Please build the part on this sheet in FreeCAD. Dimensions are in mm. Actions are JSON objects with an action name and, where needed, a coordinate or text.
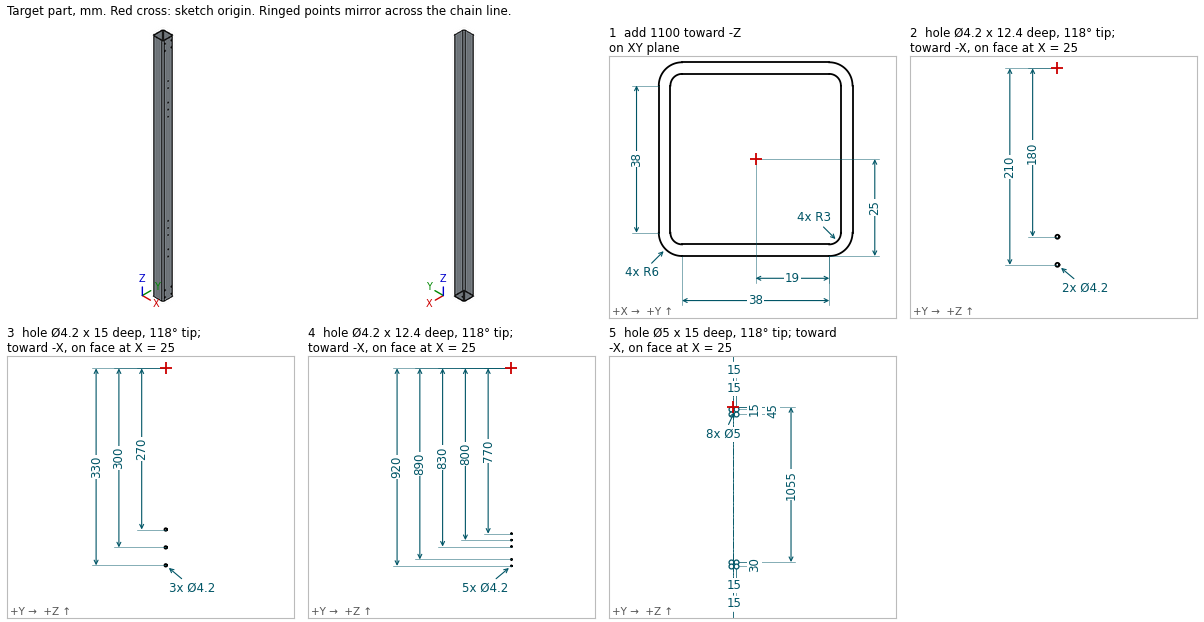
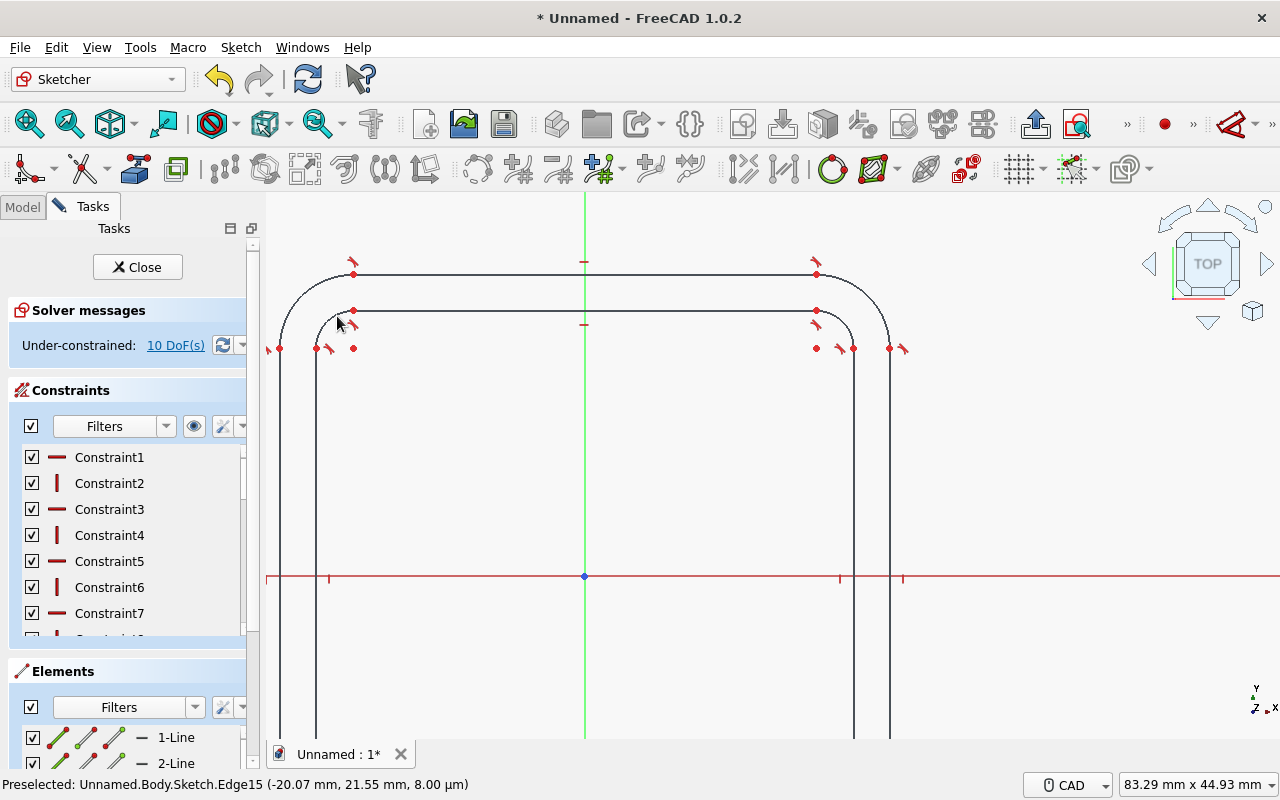
{"action": "scroll", "coordinate": [850, 330], "scroll_direction": "down", "scroll_amount": 3}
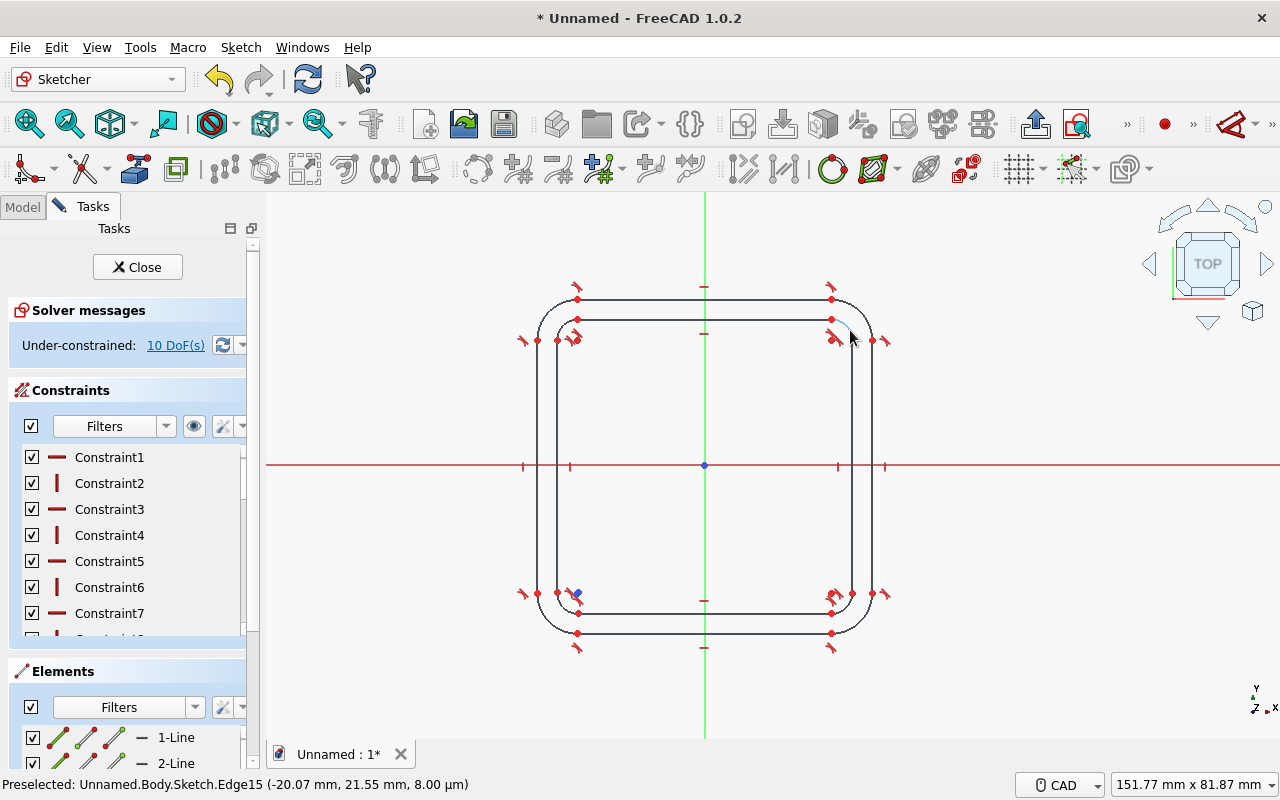
{"action": "left_click", "coordinate": [542, 612]}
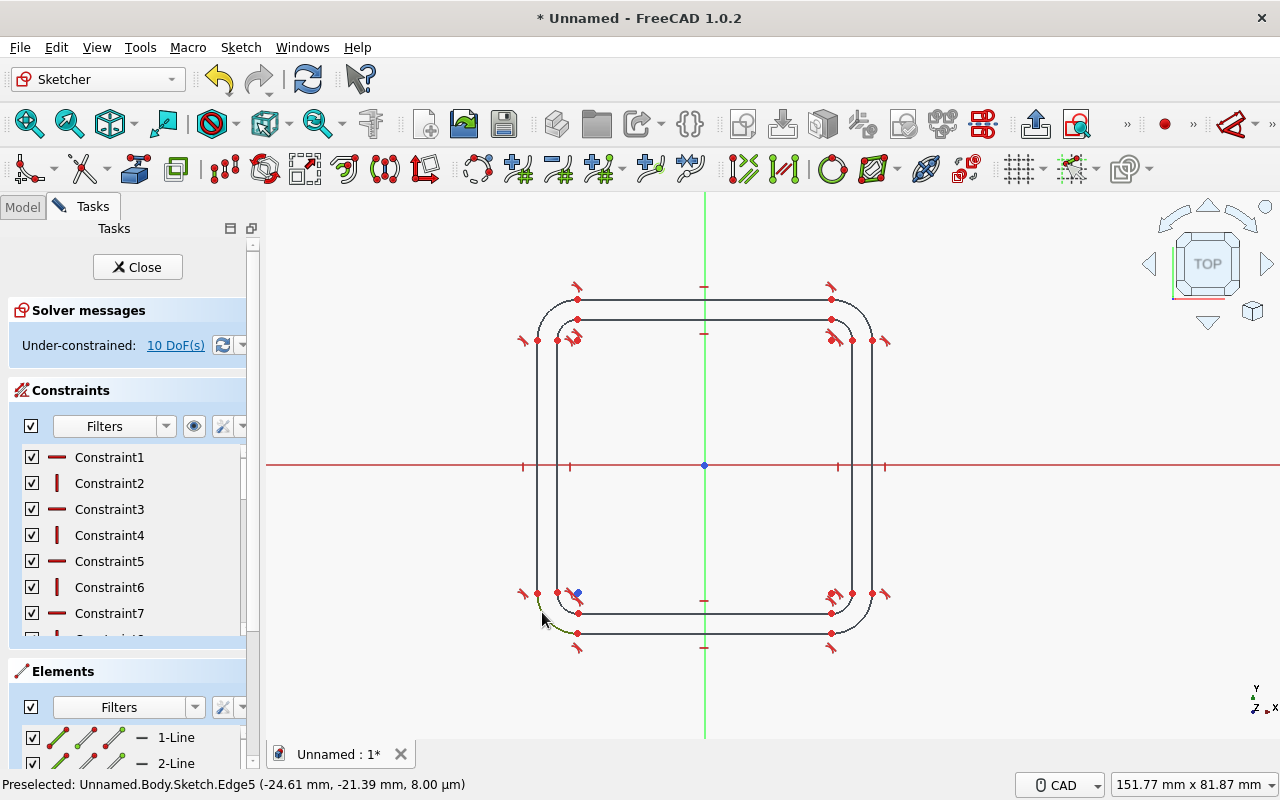
{"action": "left_click", "coordinate": [559, 304]}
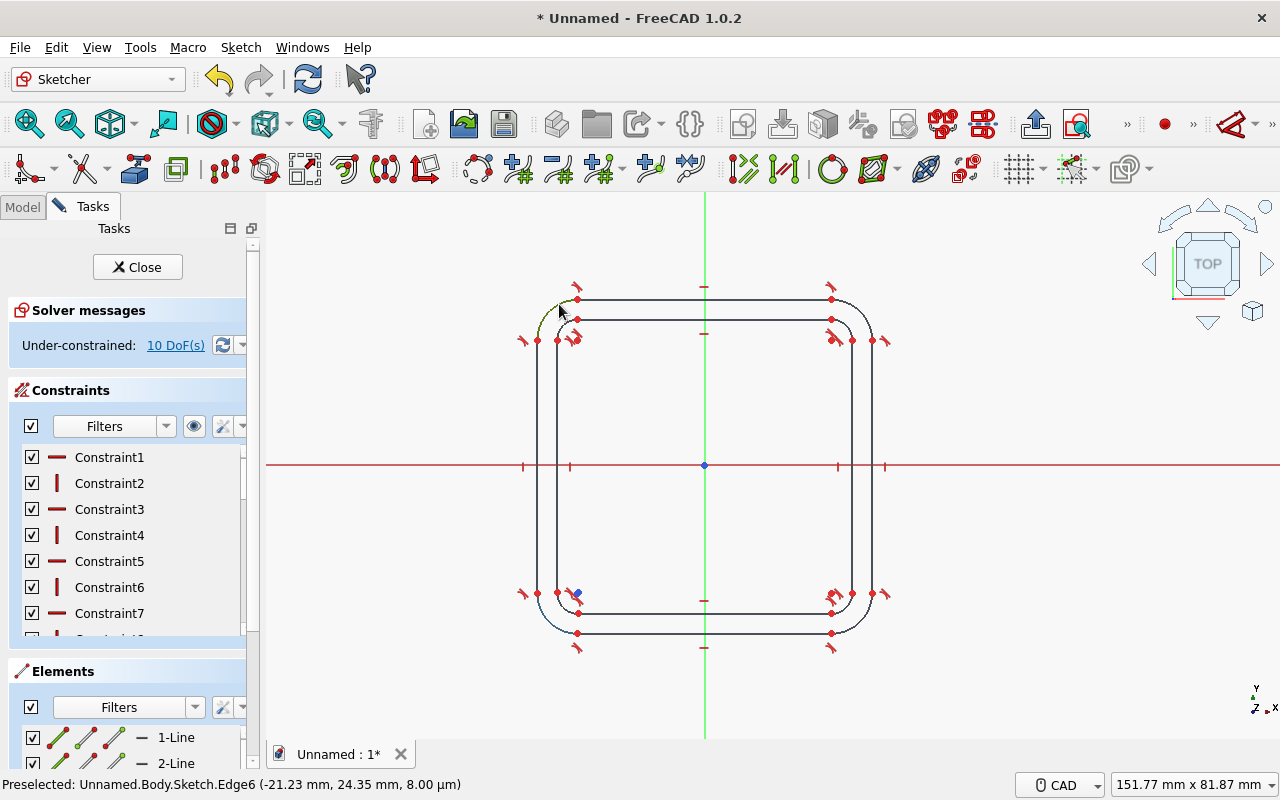
{"action": "left_click", "coordinate": [868, 322]}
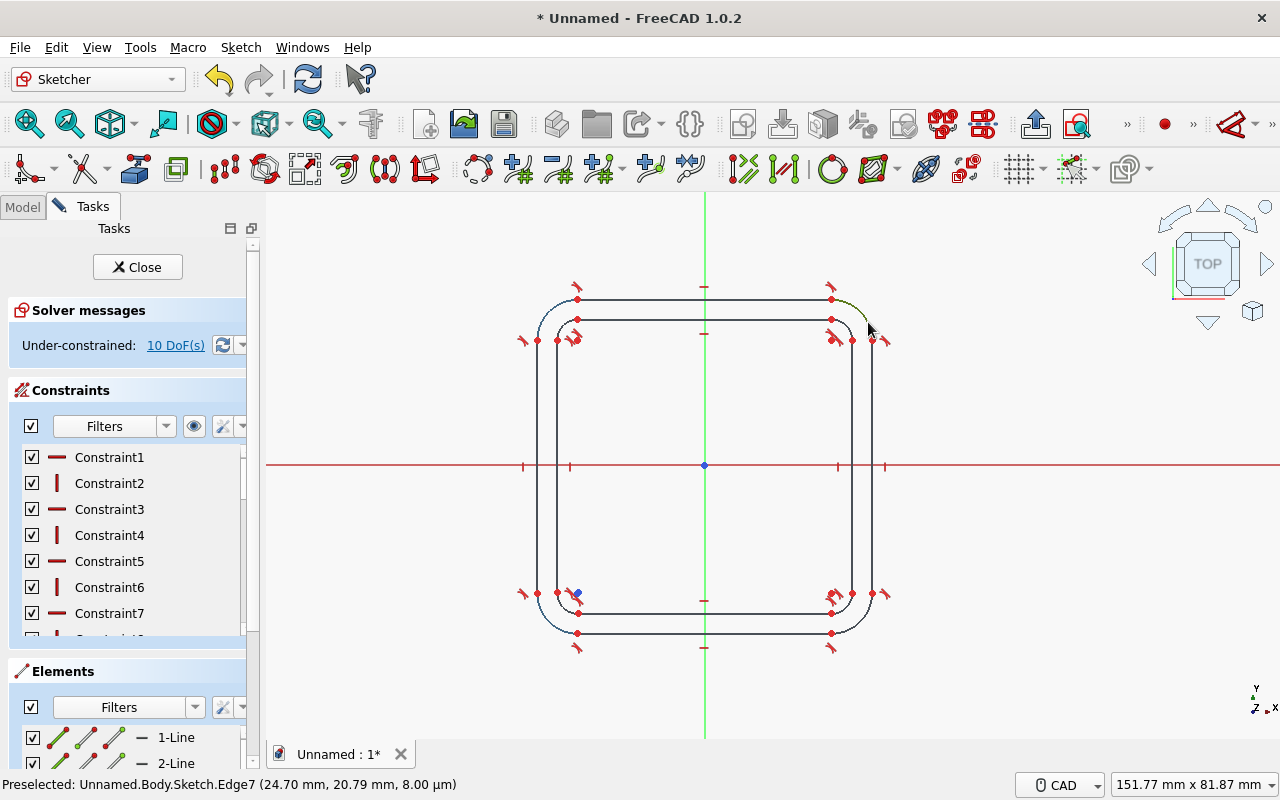
{"action": "left_click", "coordinate": [850, 629]}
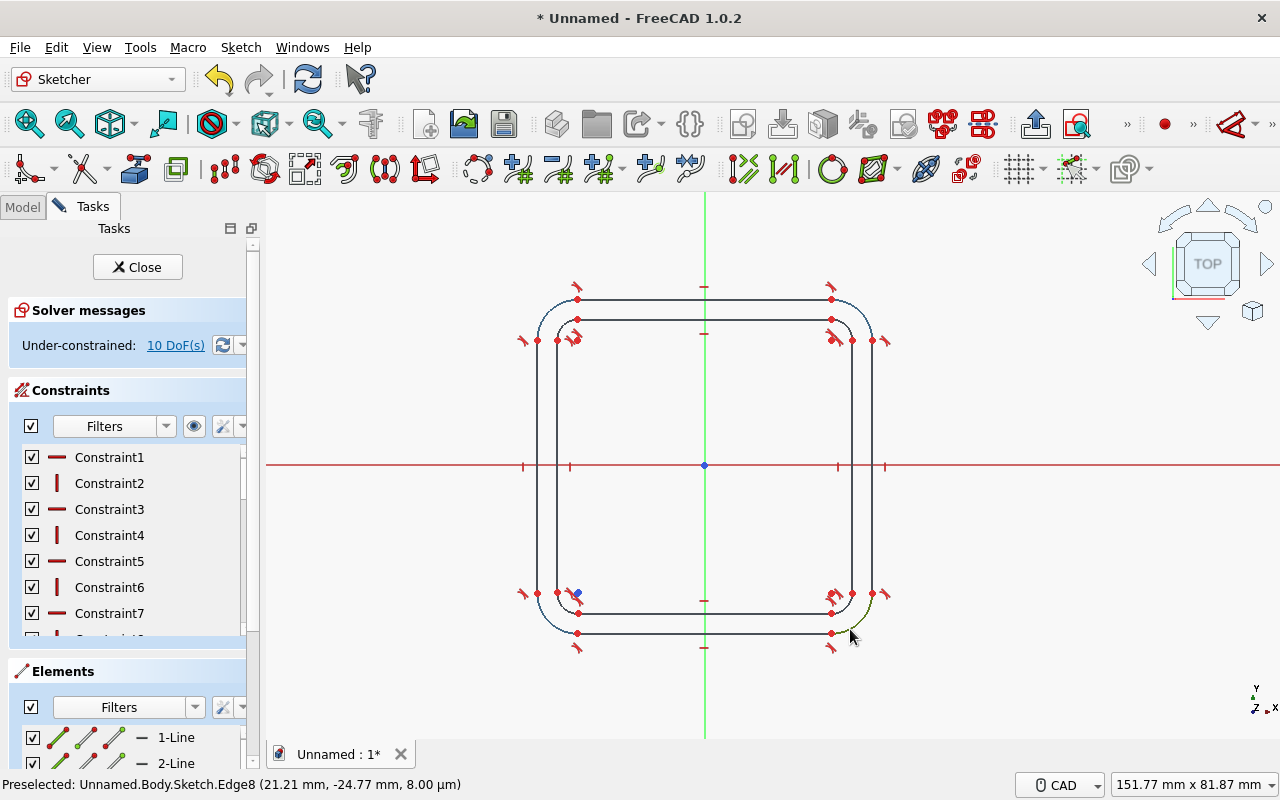
{"action": "key", "text": "e"}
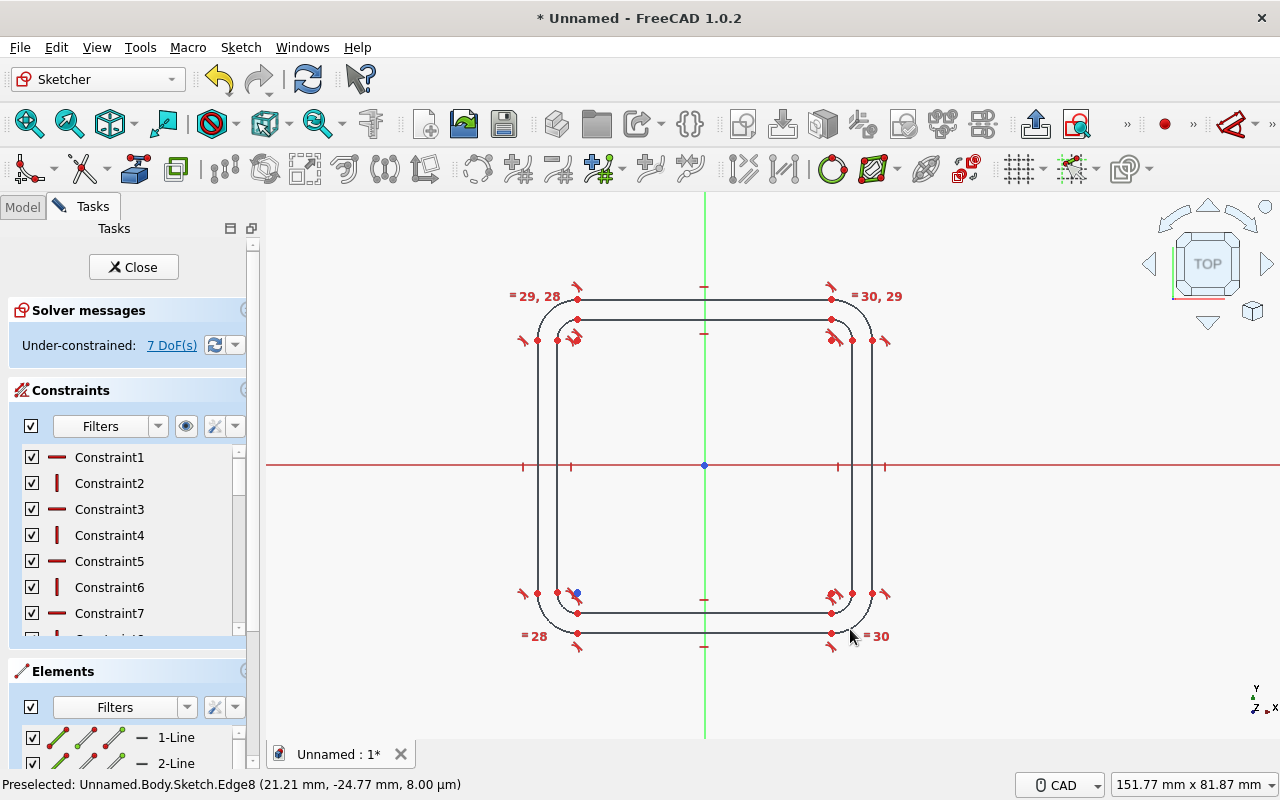
{"action": "scroll", "coordinate": [841, 611], "scroll_direction": "up", "scroll_amount": 2}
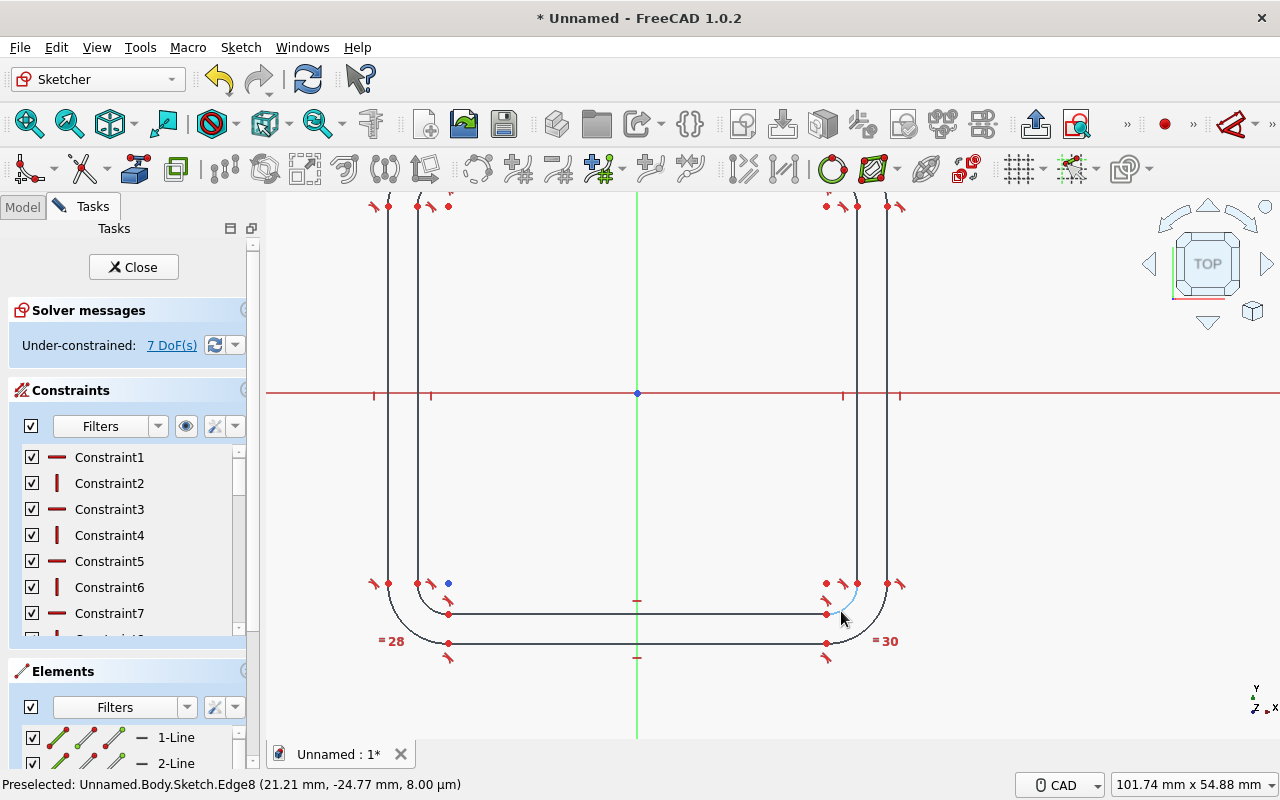
{"action": "left_click", "coordinate": [841, 611]}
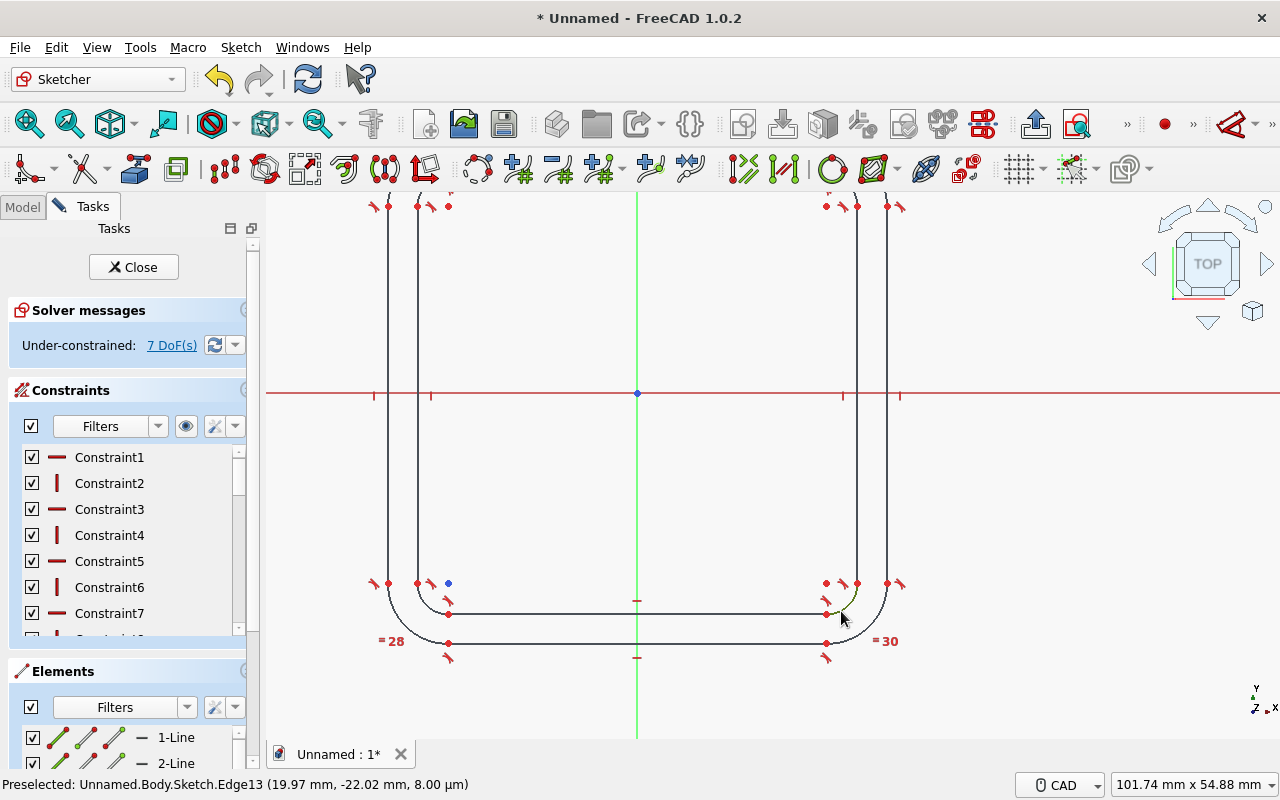
{"action": "left_click", "coordinate": [421, 598]}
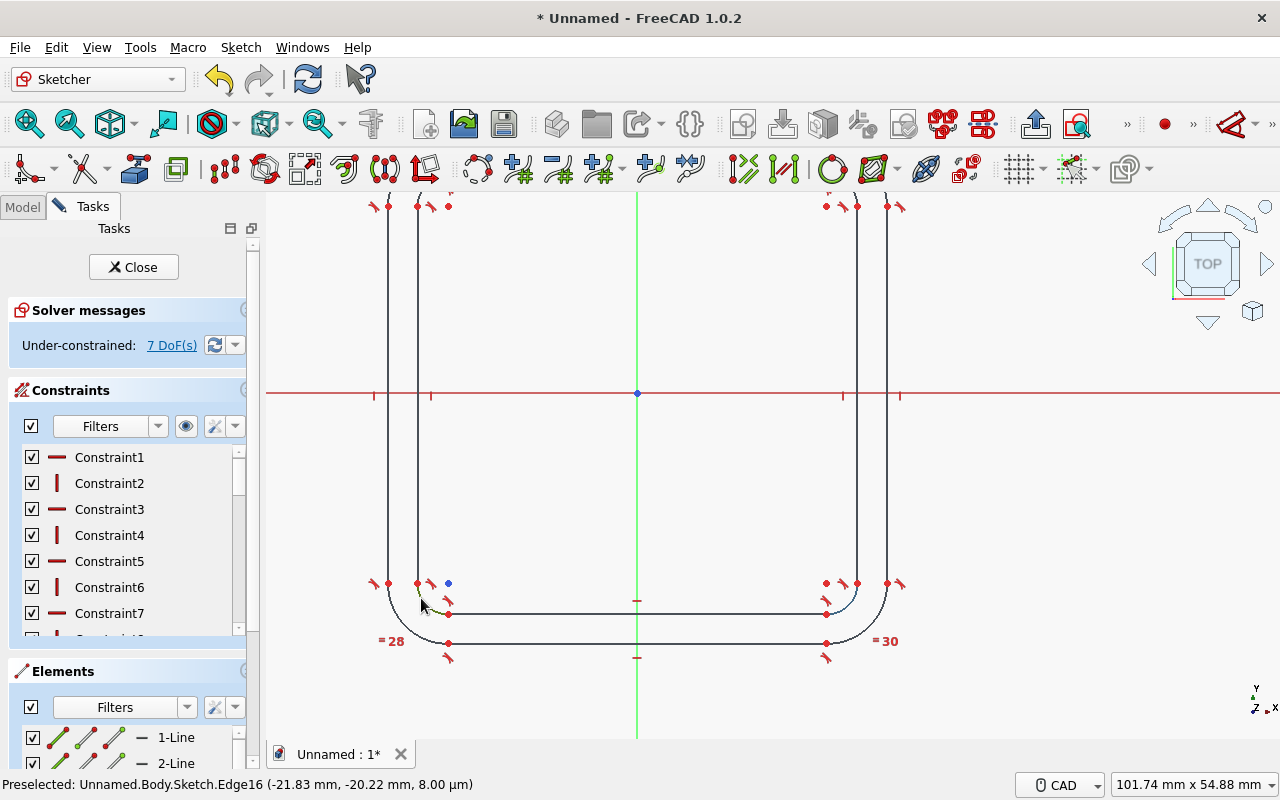
{"action": "key", "text": "e"}